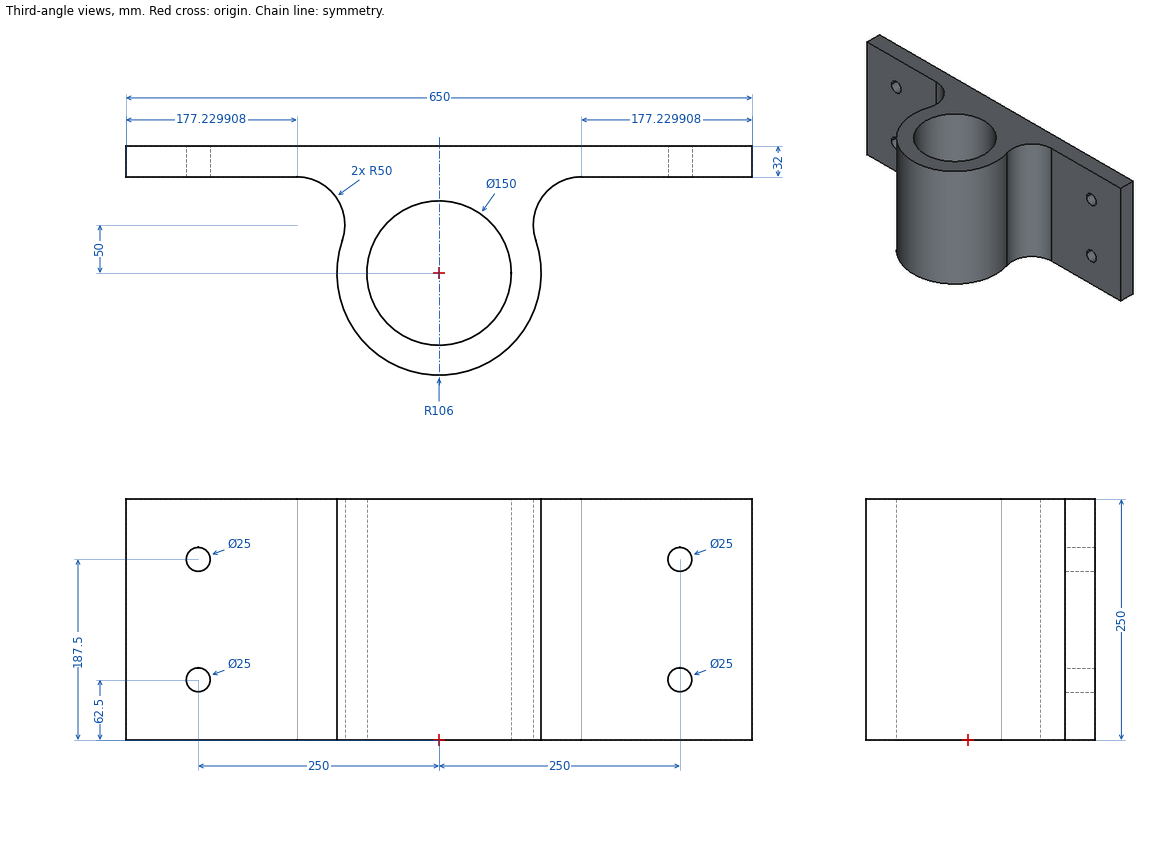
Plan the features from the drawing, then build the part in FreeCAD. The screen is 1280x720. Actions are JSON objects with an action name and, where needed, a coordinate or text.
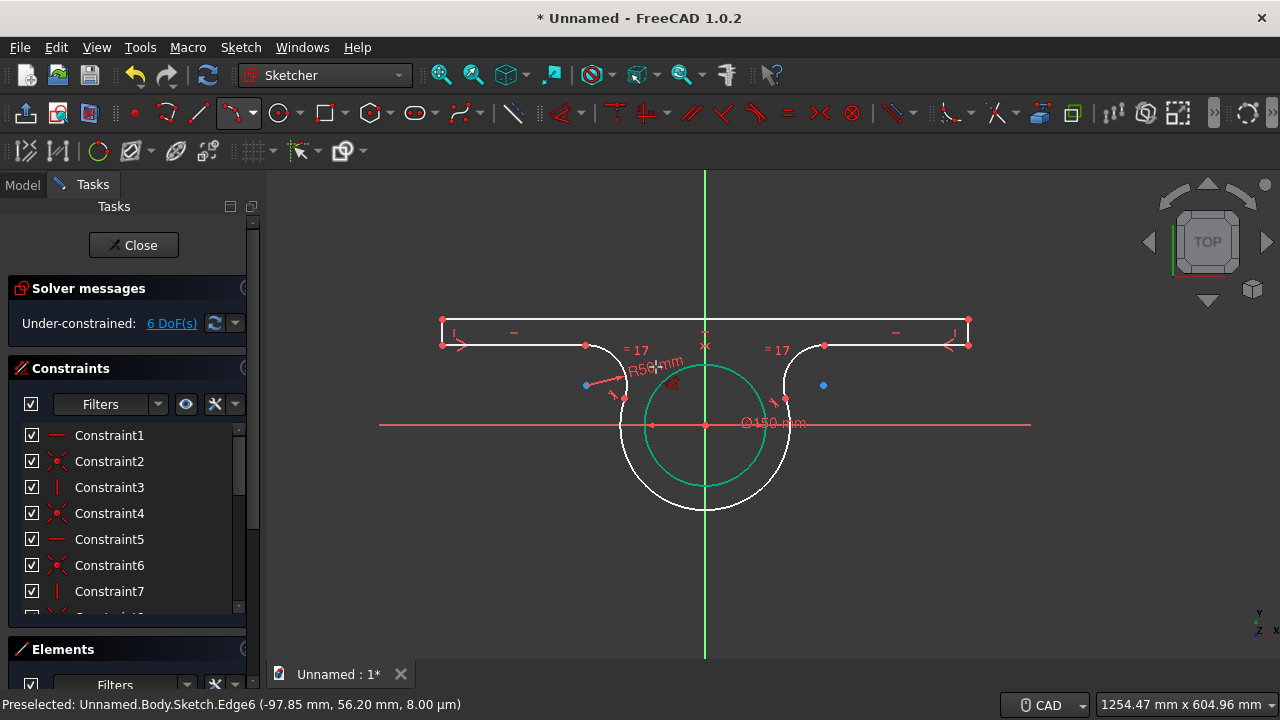
{"action": "left_click", "coordinate": [647, 487]}
{"action": "left_click", "coordinate": [625, 510]}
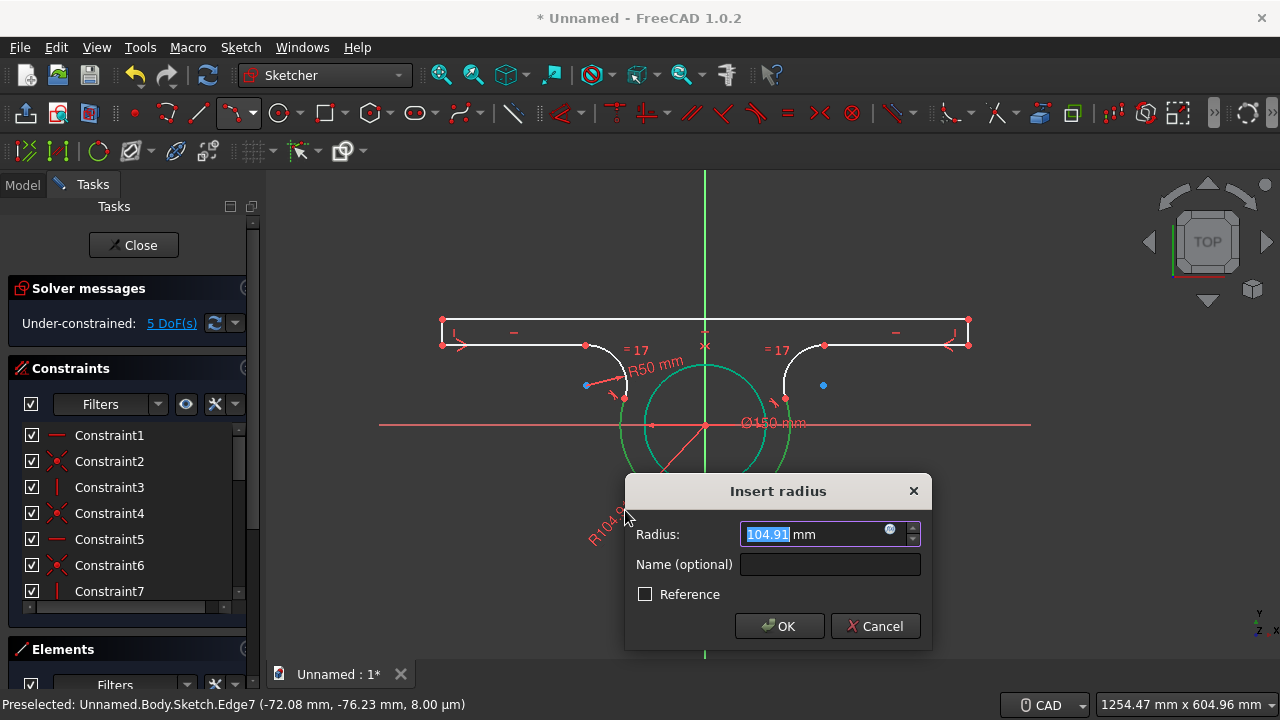
{"action": "type", "text": "106"}
{"action": "key", "text": "Return"}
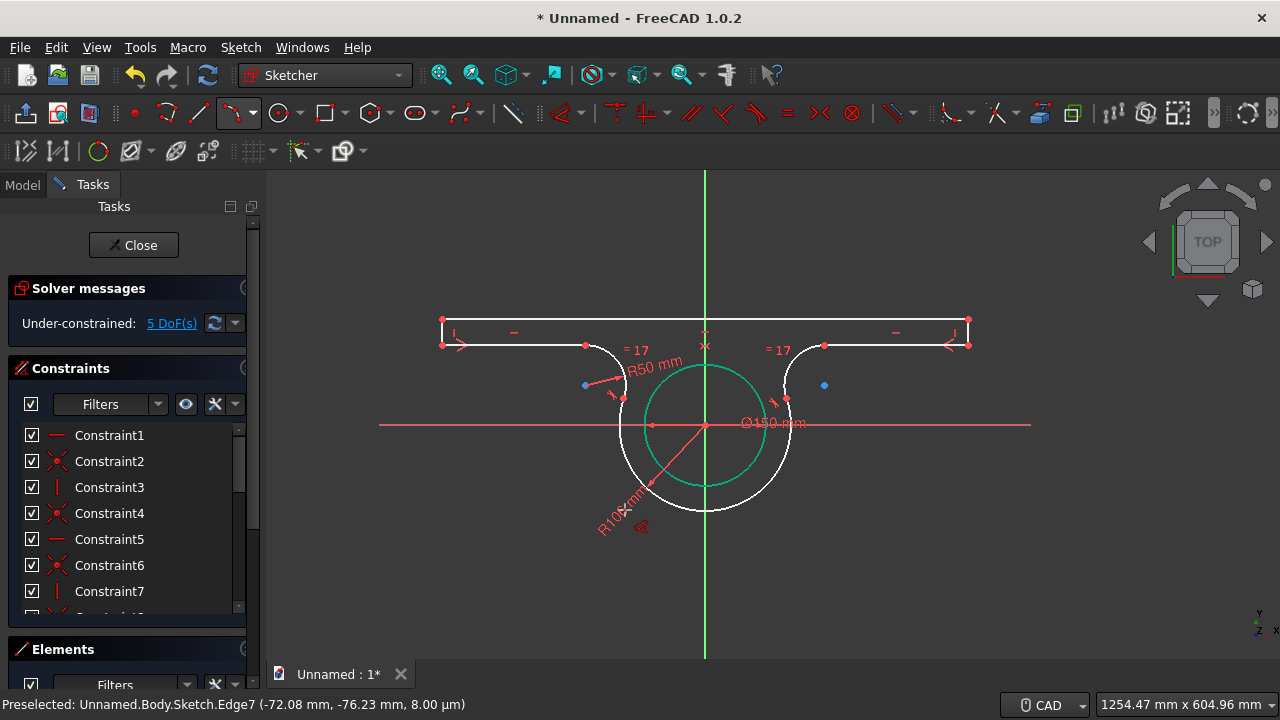
{"action": "scroll", "coordinate": [968, 335], "scroll_direction": "up", "scroll_amount": 3}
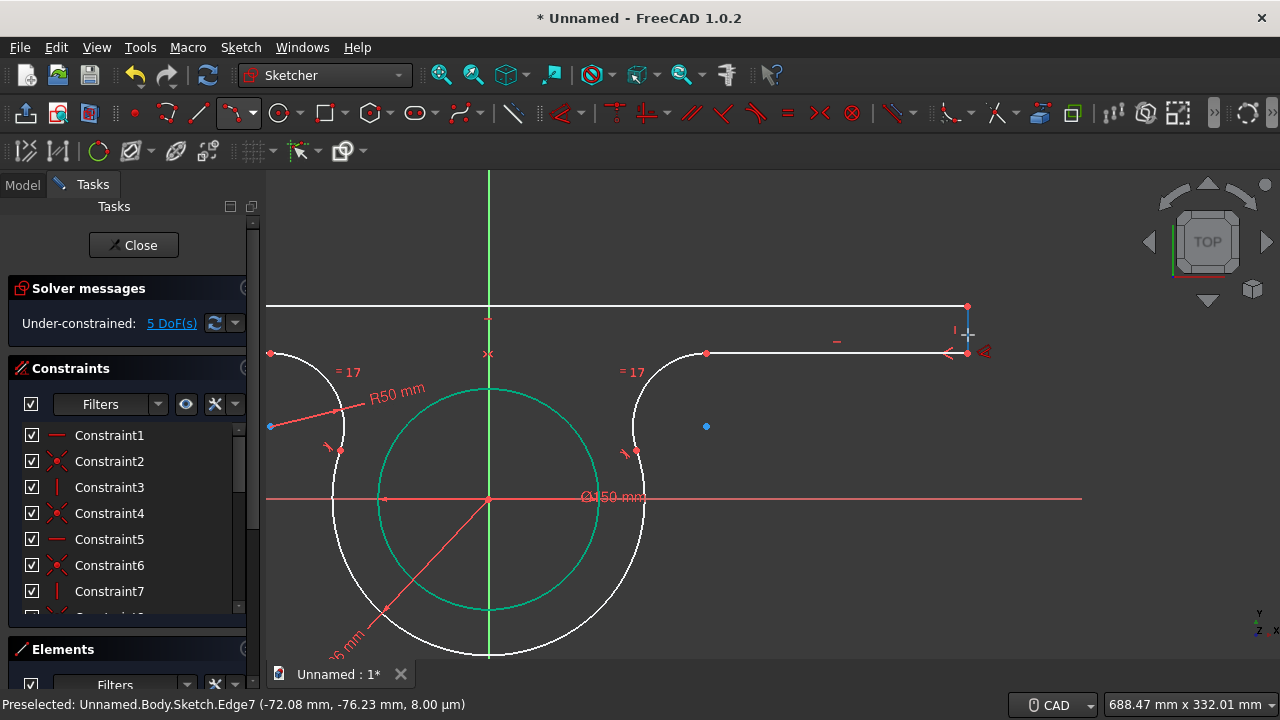
{"action": "left_click", "coordinate": [968, 334]}
{"action": "left_click", "coordinate": [1002, 330]}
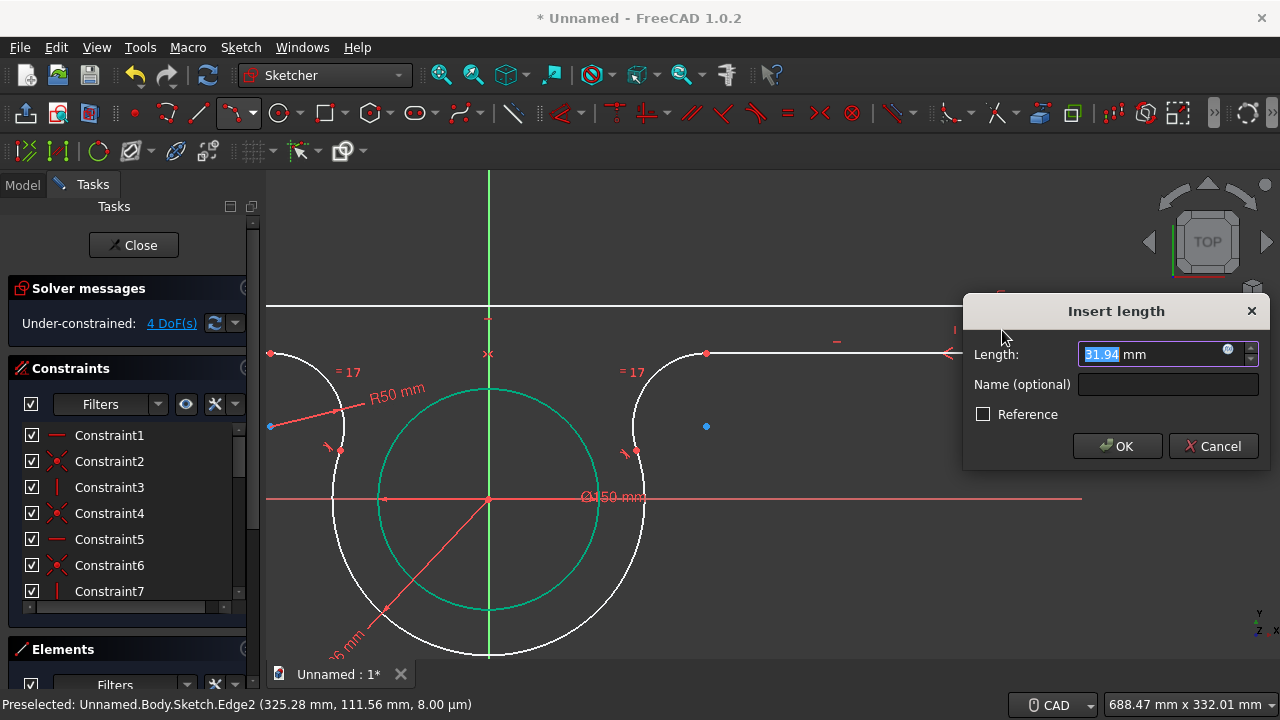
{"action": "type", "text": "32"}
{"action": "key", "text": "Return"}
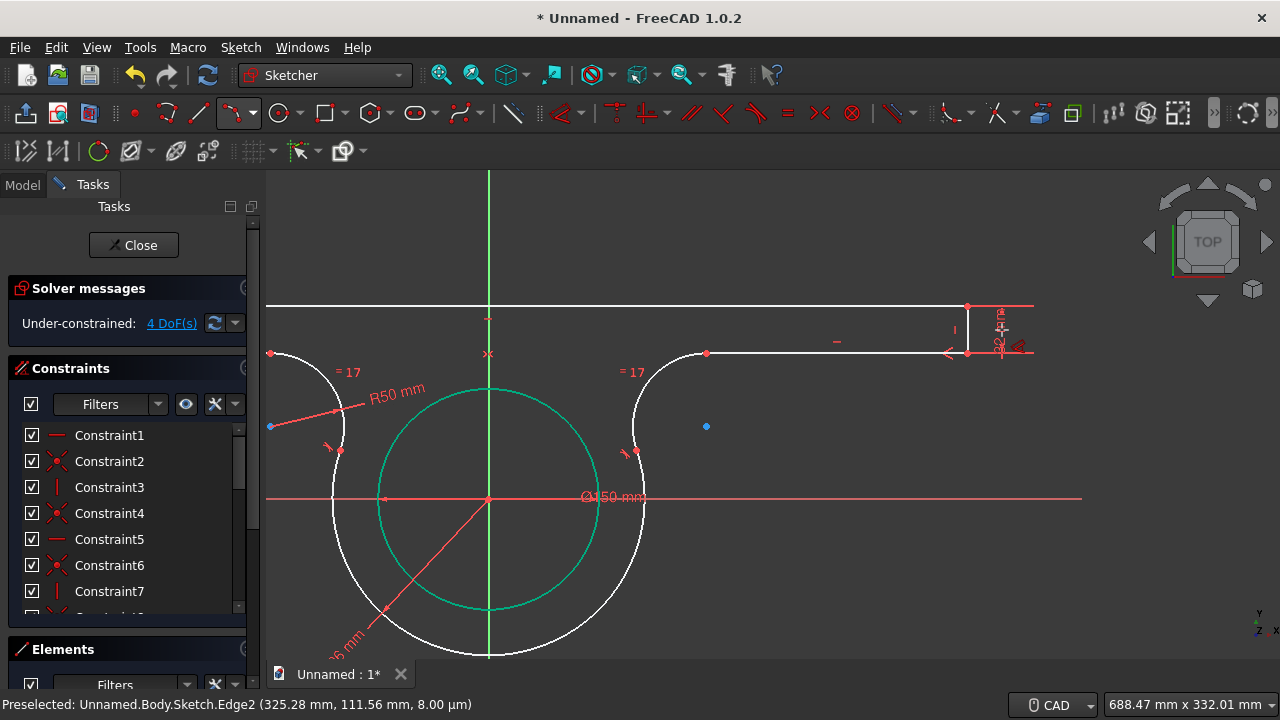
{"action": "left_click", "coordinate": [680, 306]}
{"action": "left_click", "coordinate": [631, 272]}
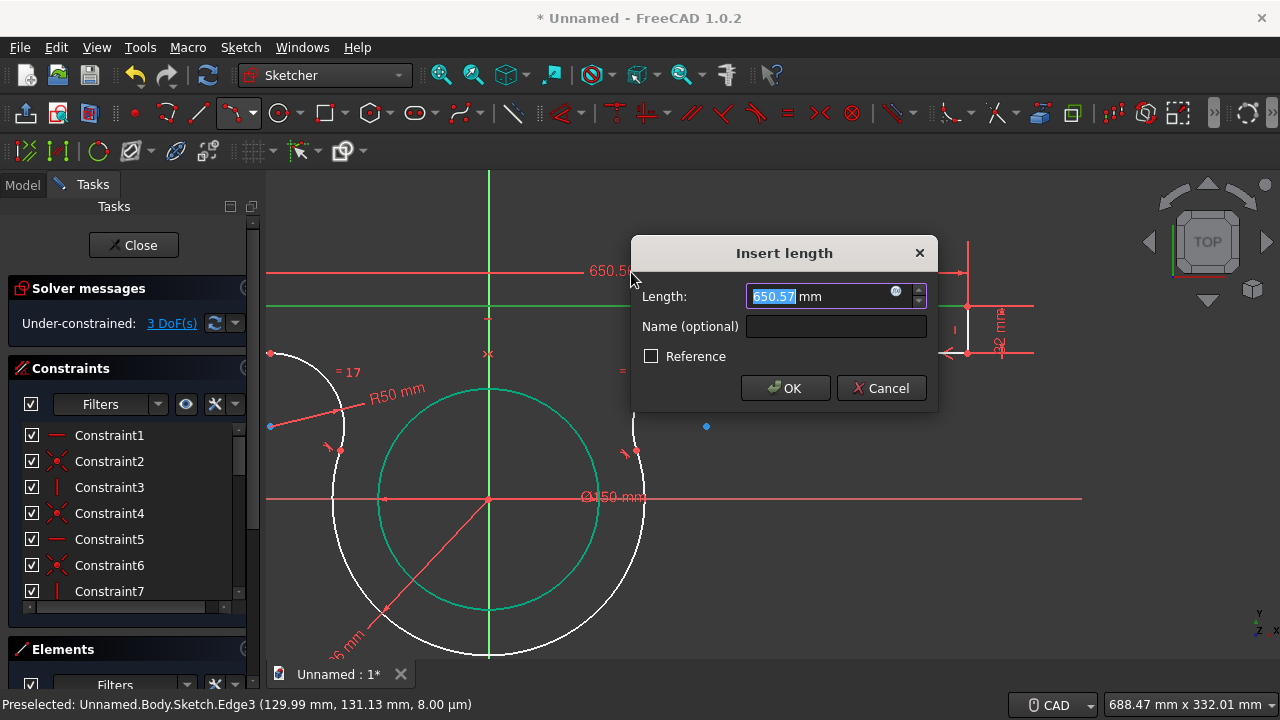
{"action": "type", "text": "650"}
{"action": "key", "text": "Return"}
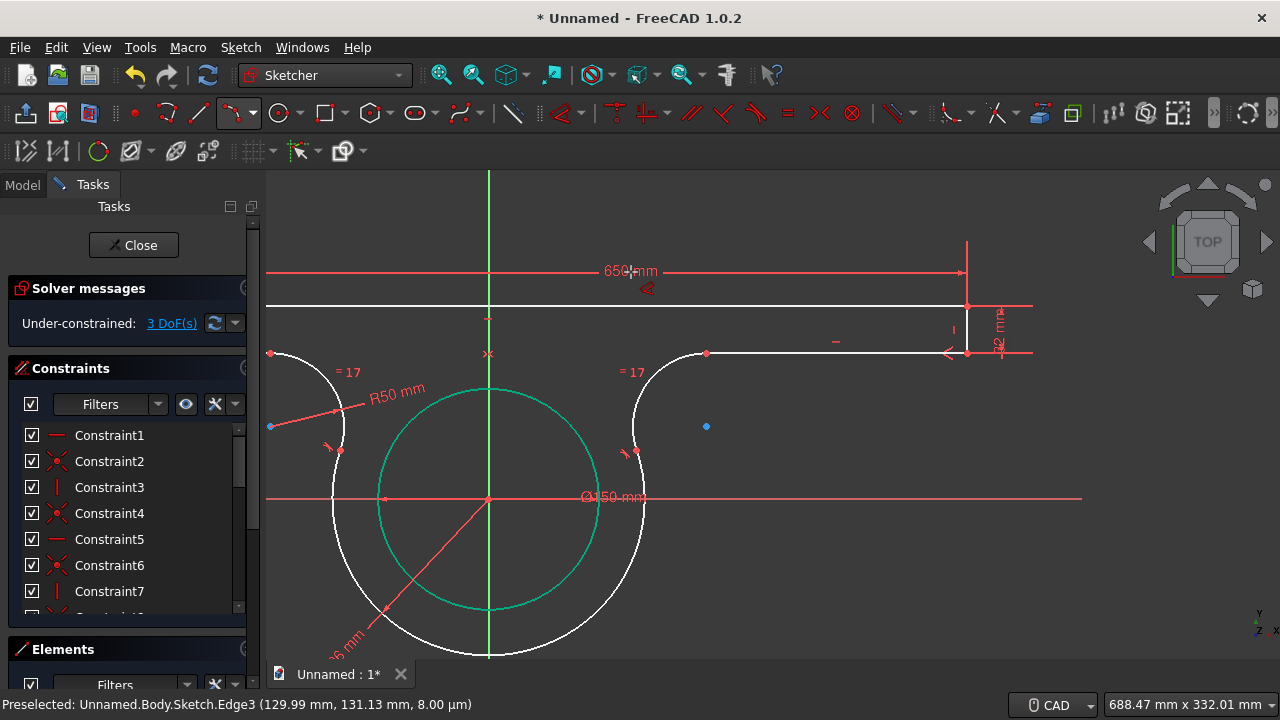
{"action": "scroll", "coordinate": [967, 335], "scroll_direction": "down", "scroll_amount": 3}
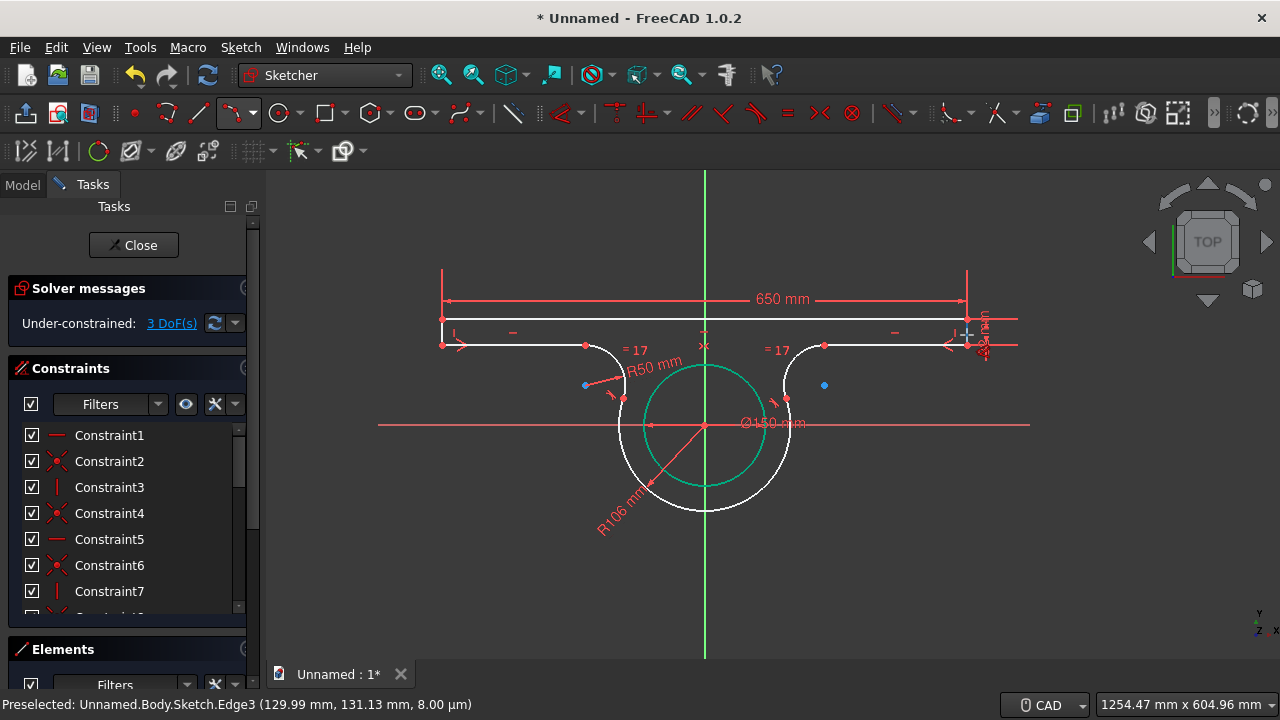
{"action": "left_click", "coordinate": [585, 386]}
{"action": "left_click", "coordinate": [551, 405]}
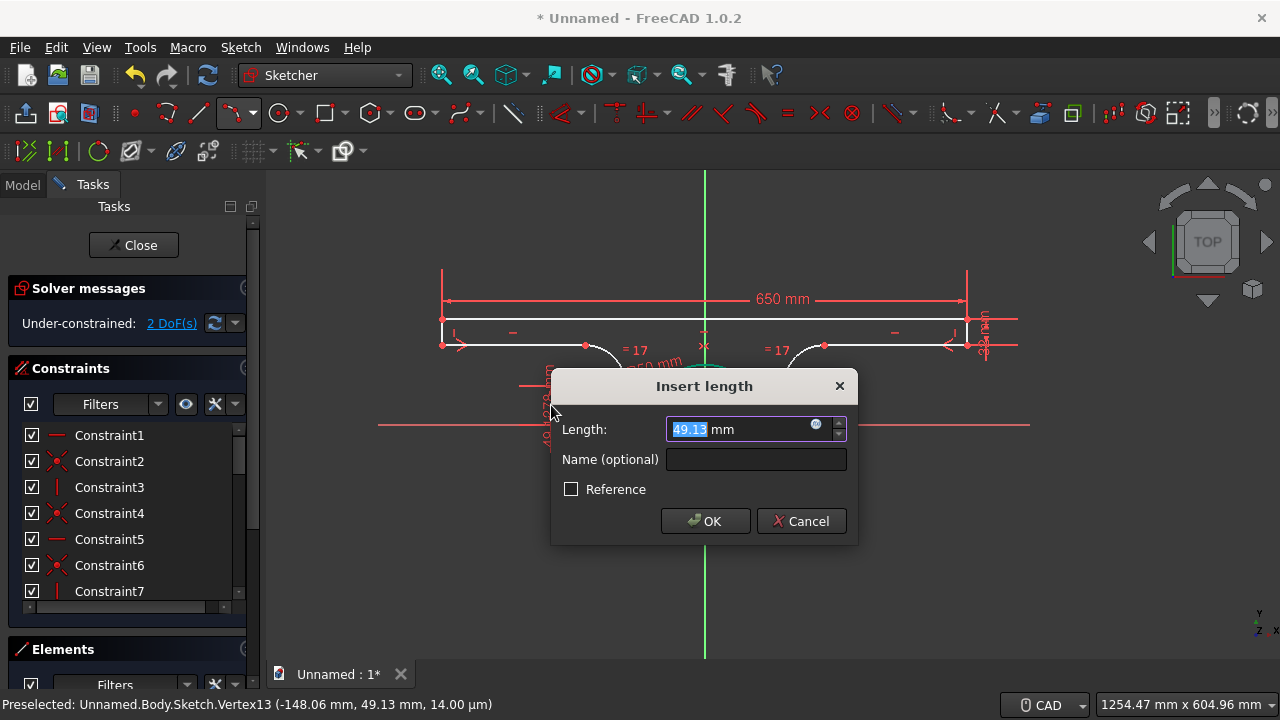
{"action": "type", "text": "50"}
{"action": "key", "text": "Return"}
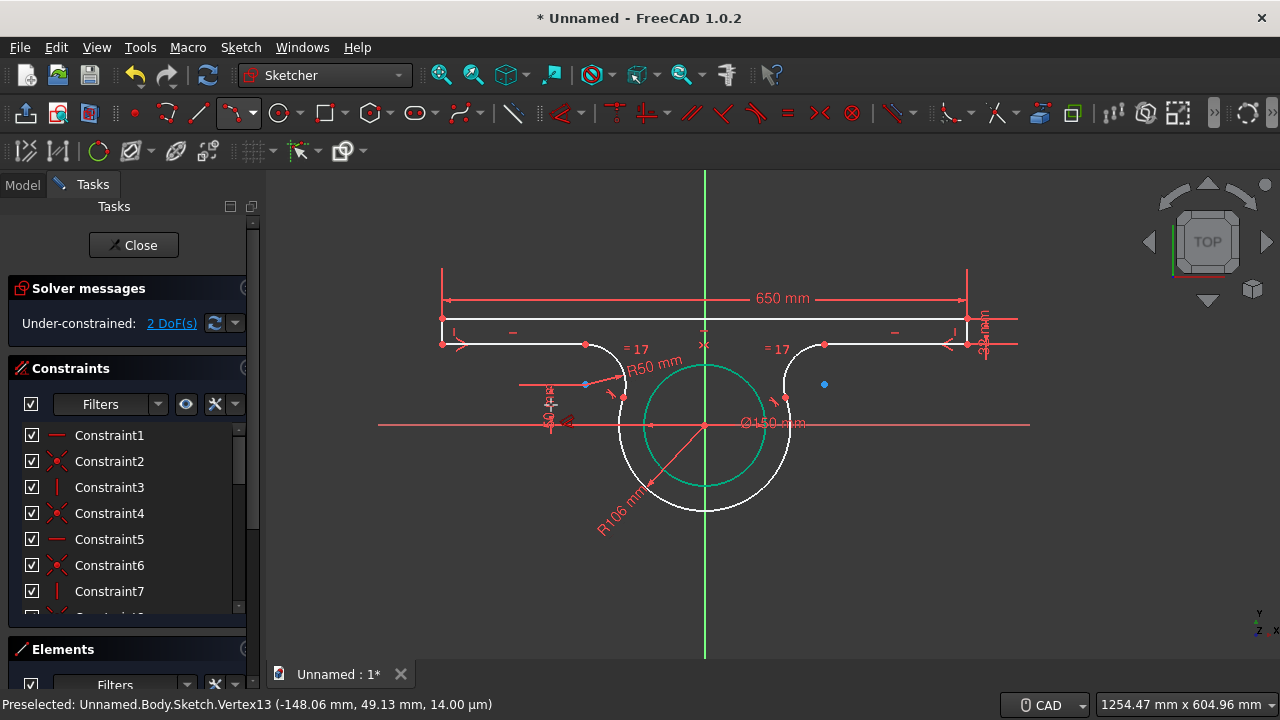
{"action": "left_click", "coordinate": [867, 344]}
{"action": "left_click", "coordinate": [896, 378]}